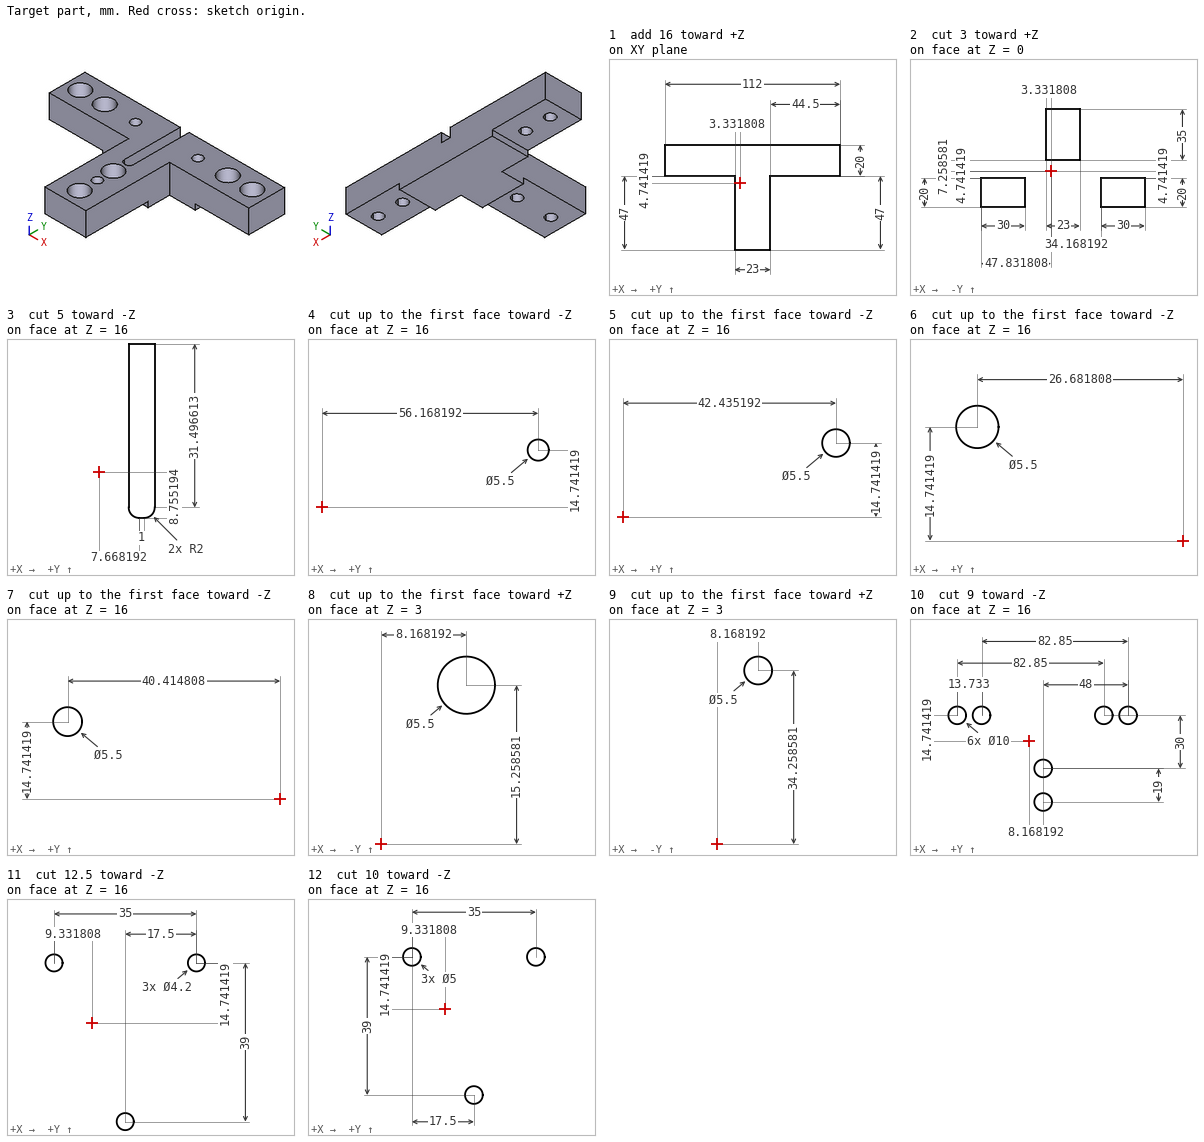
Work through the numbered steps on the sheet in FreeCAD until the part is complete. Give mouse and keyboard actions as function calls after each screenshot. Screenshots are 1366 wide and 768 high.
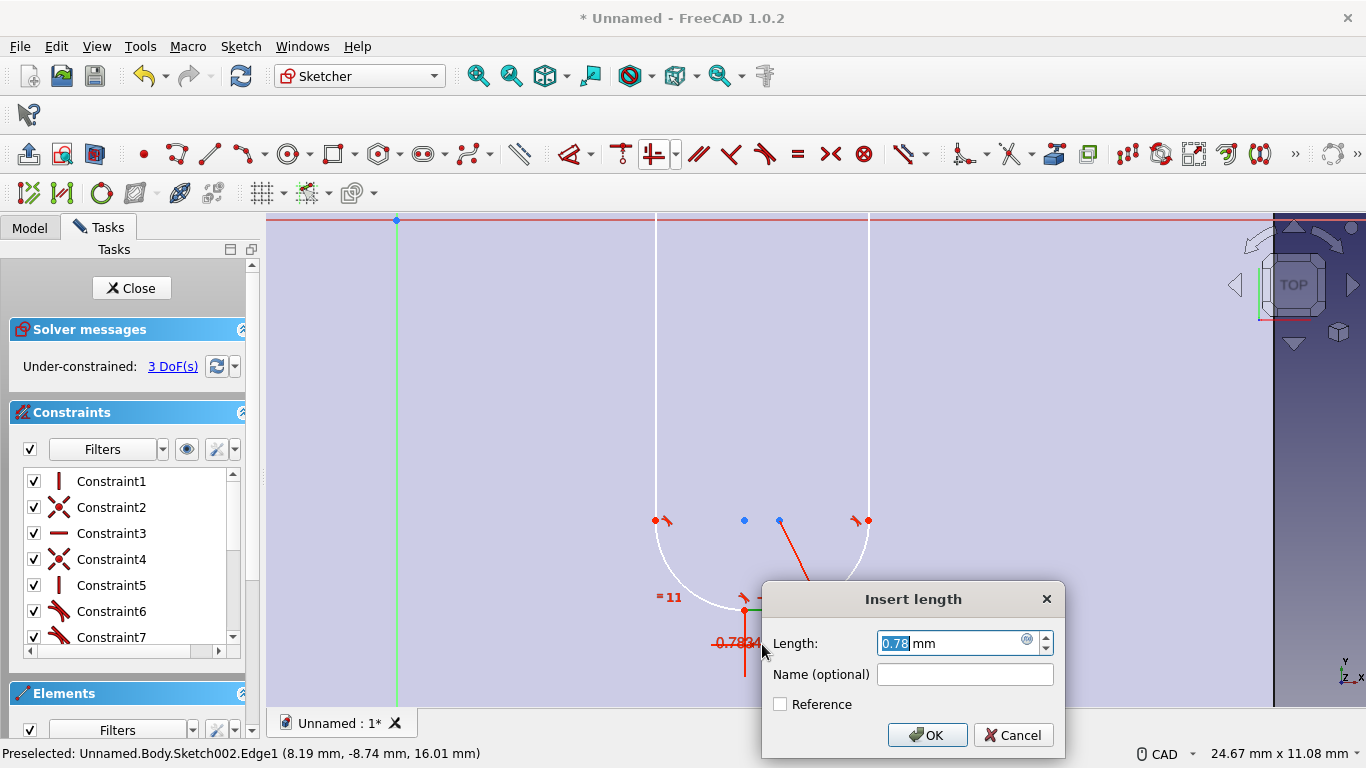
text(1)
key(Return)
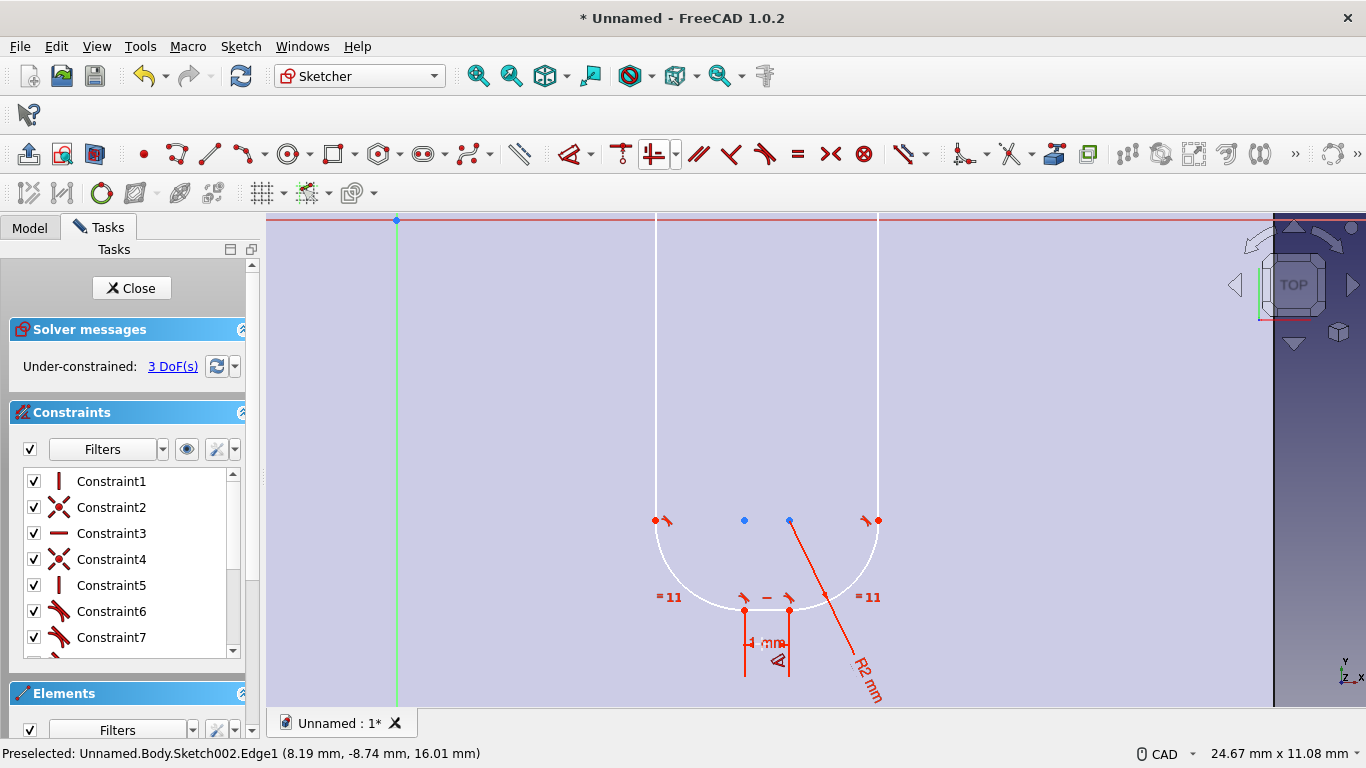
click(878, 241)
click(912, 381)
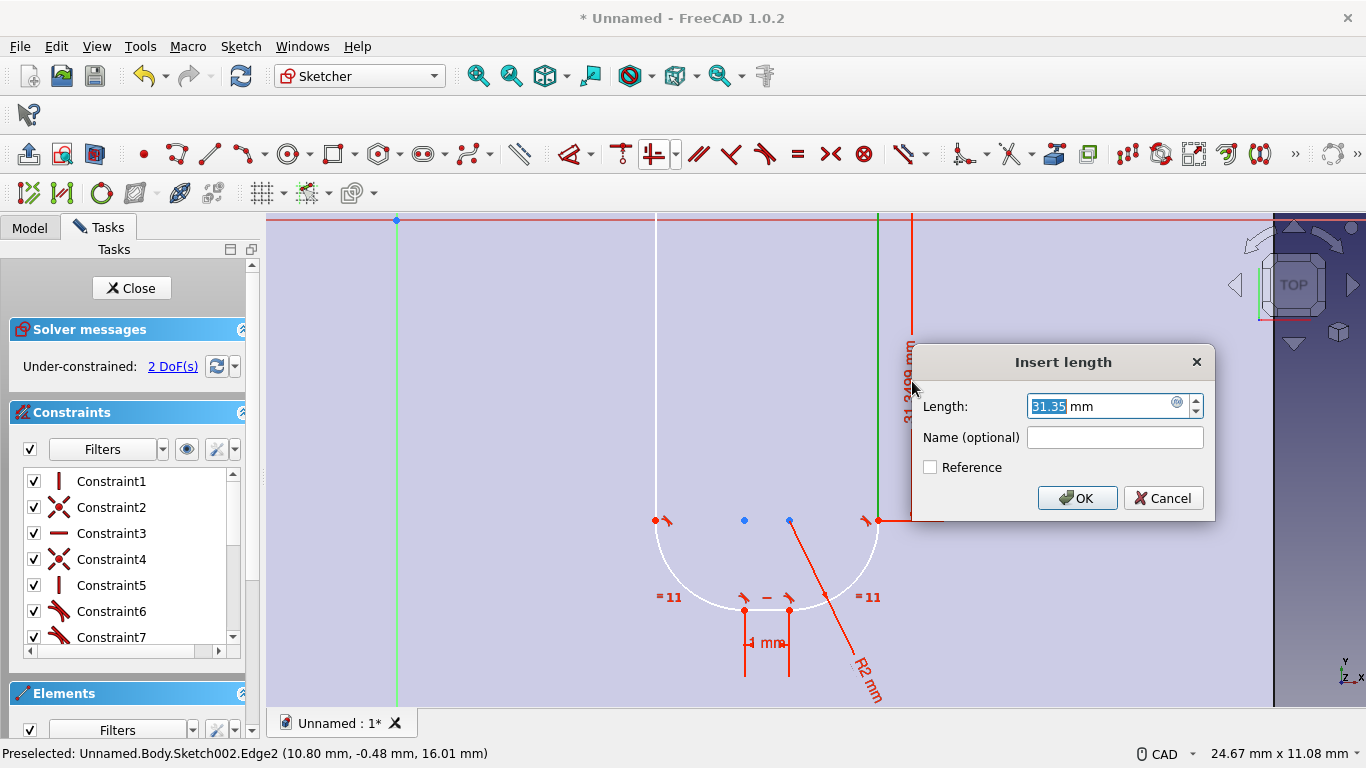
text(31.496613)
key(Return)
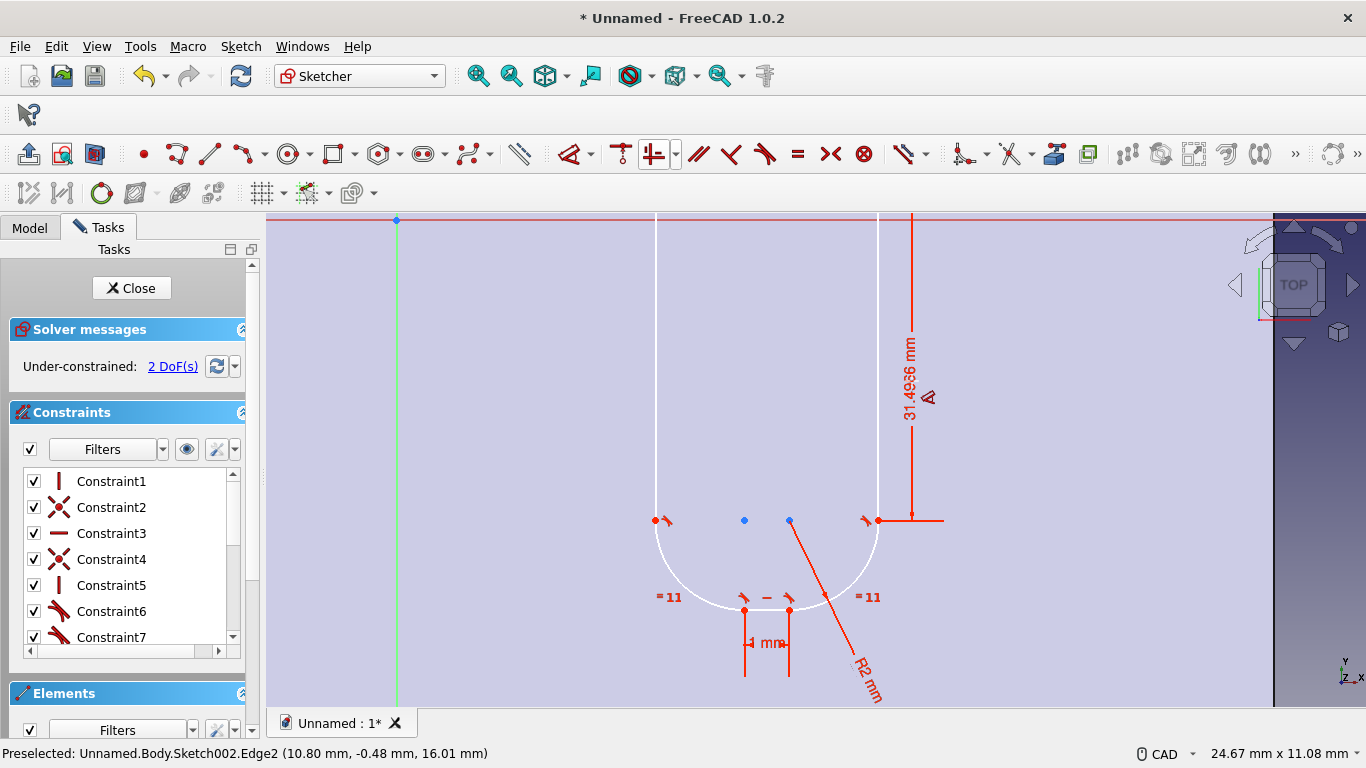
scroll(776, 611, down, 8)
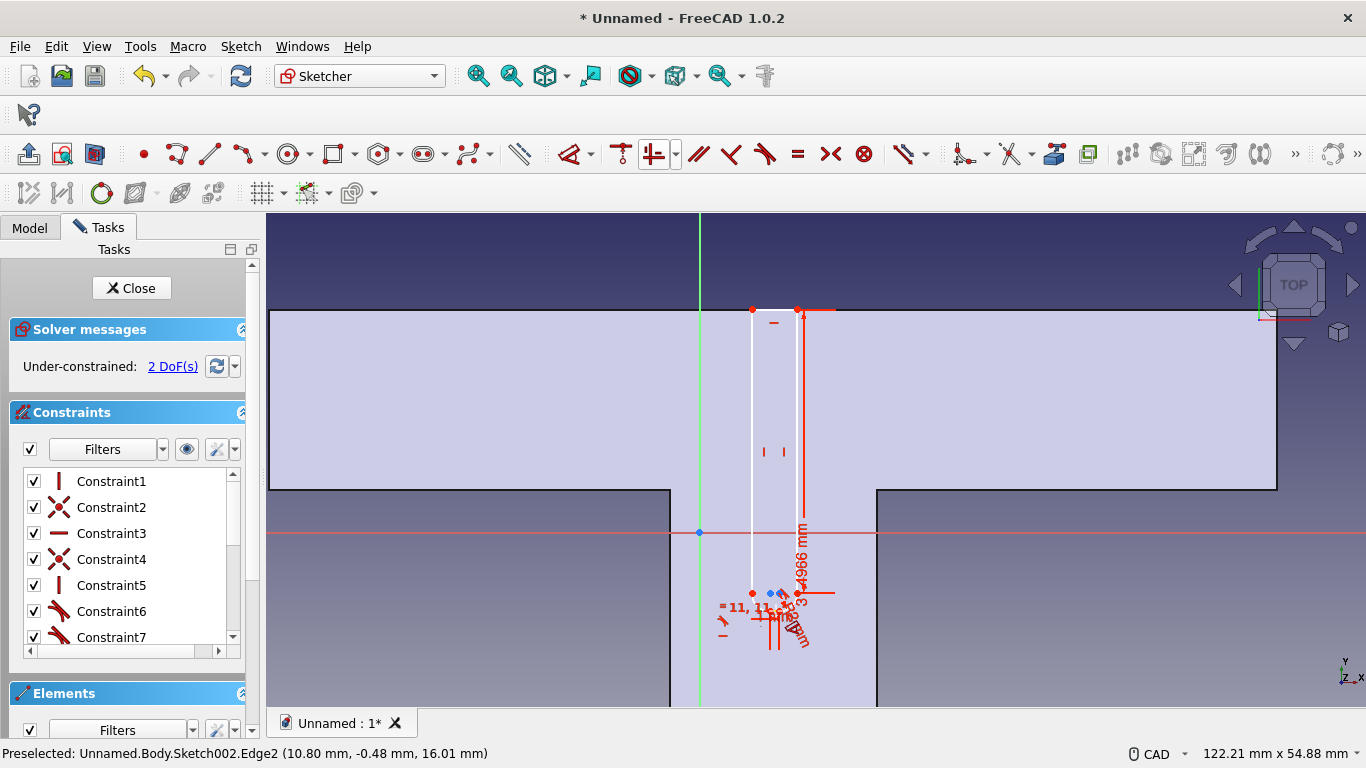
scroll(770, 611, up, 2)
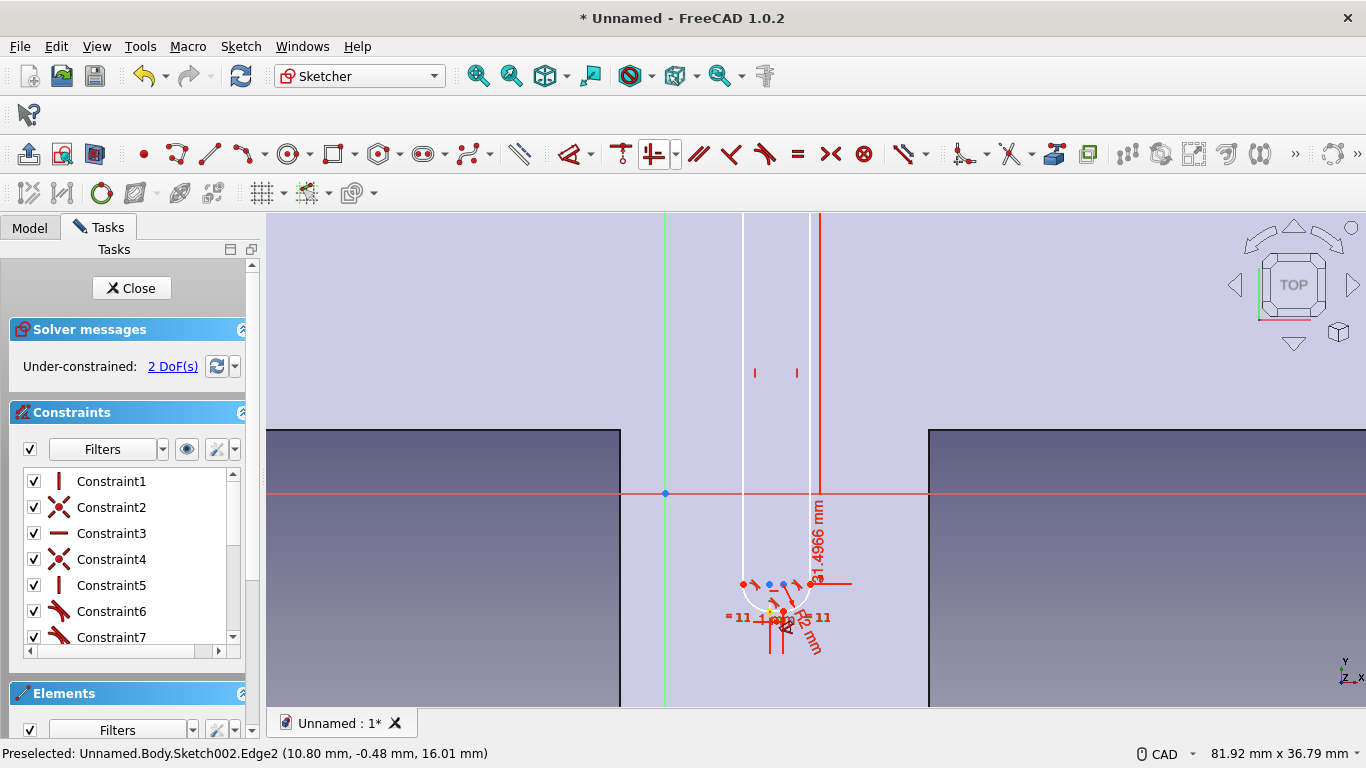
click(770, 611)
click(717, 645)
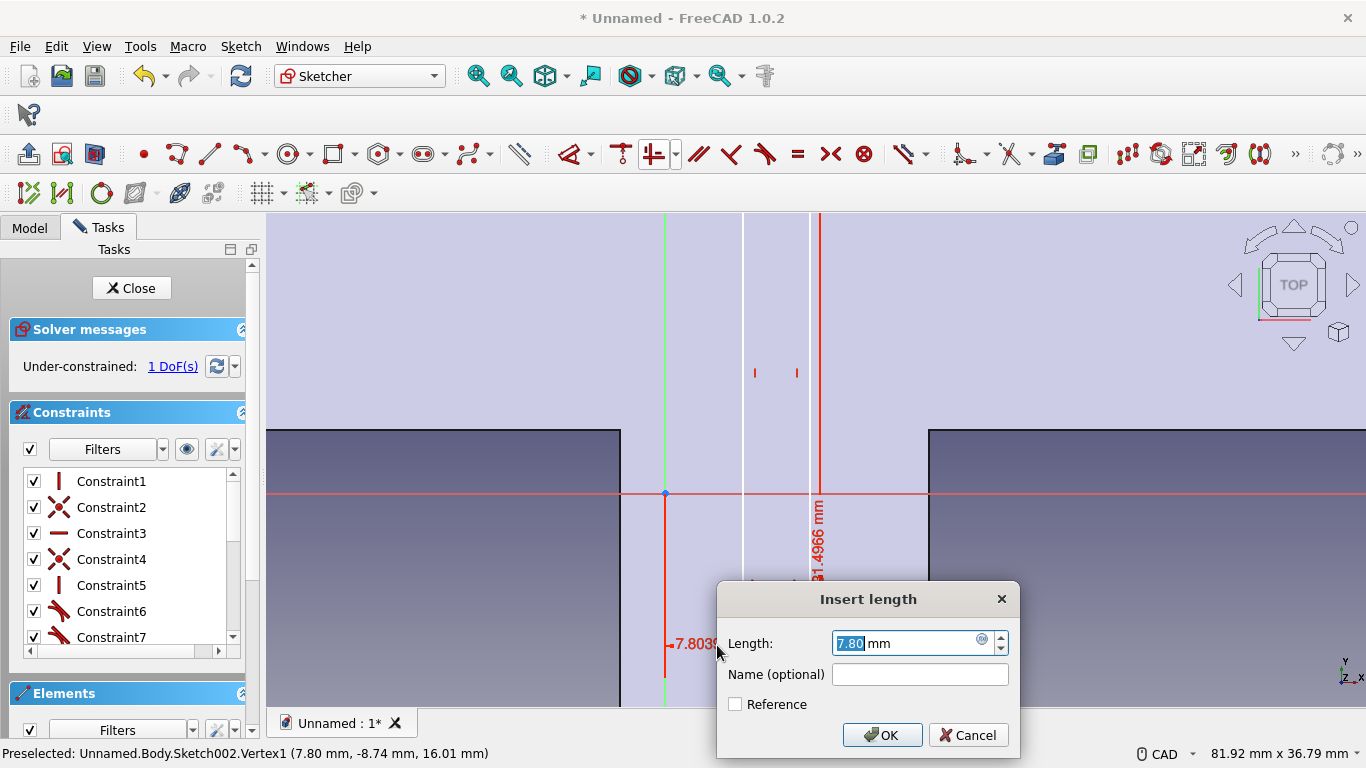
text(7.668192)
key(Return)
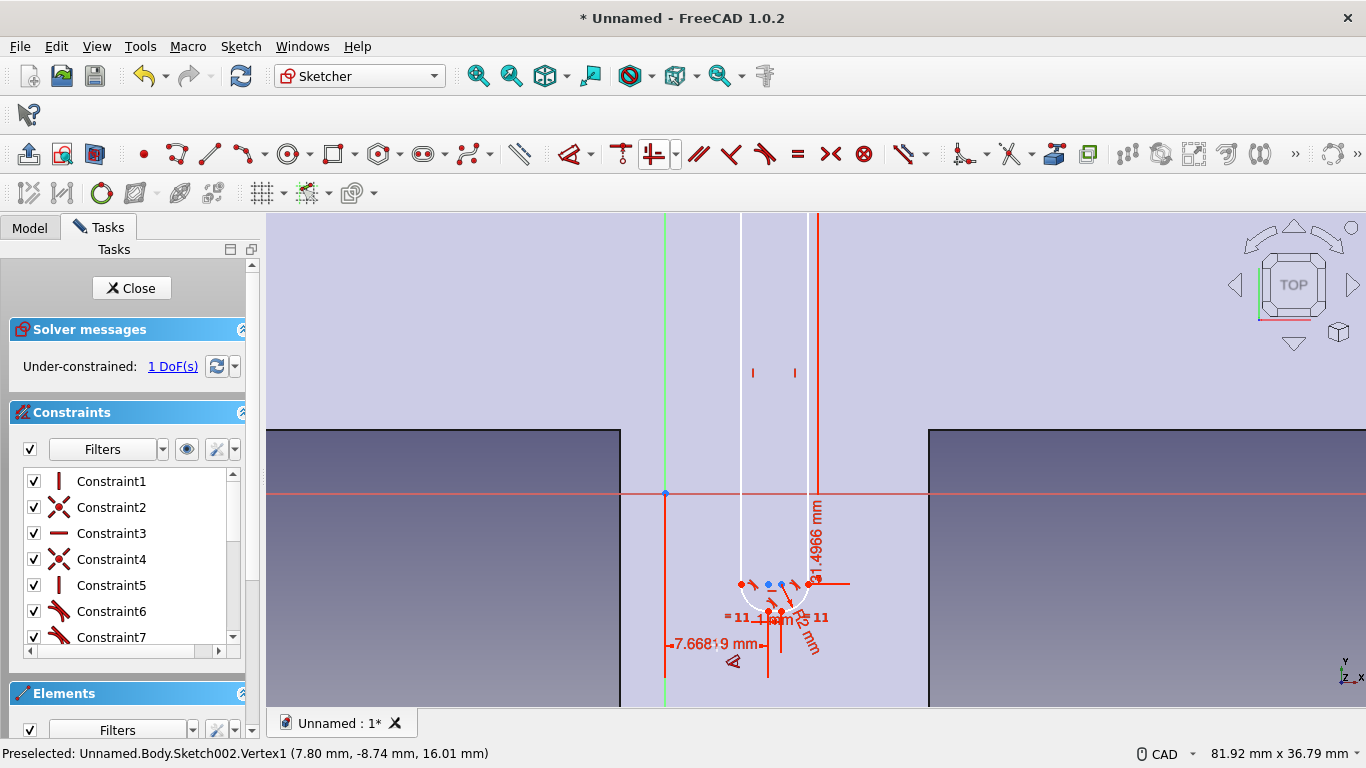
click(768, 611)
click(631, 553)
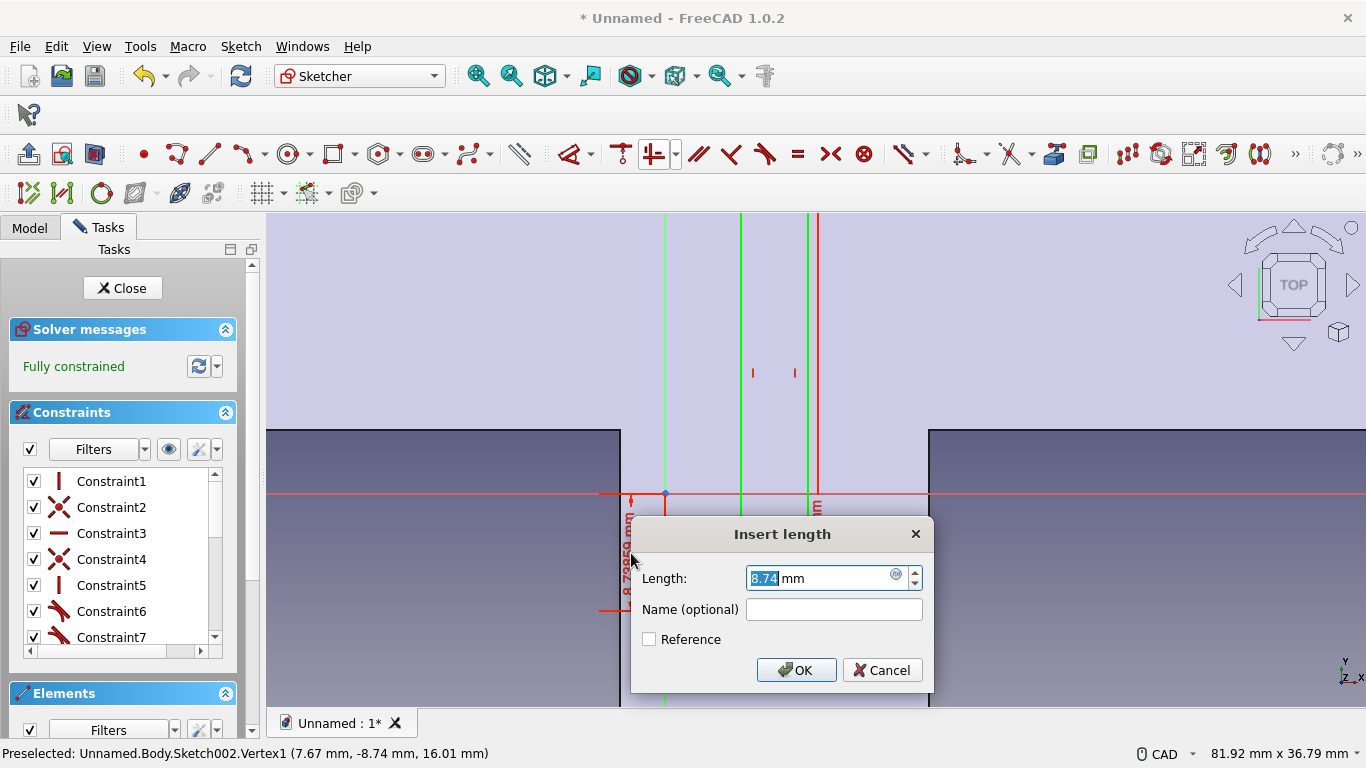
text(8.755194)
key(Return)
key(Escape)